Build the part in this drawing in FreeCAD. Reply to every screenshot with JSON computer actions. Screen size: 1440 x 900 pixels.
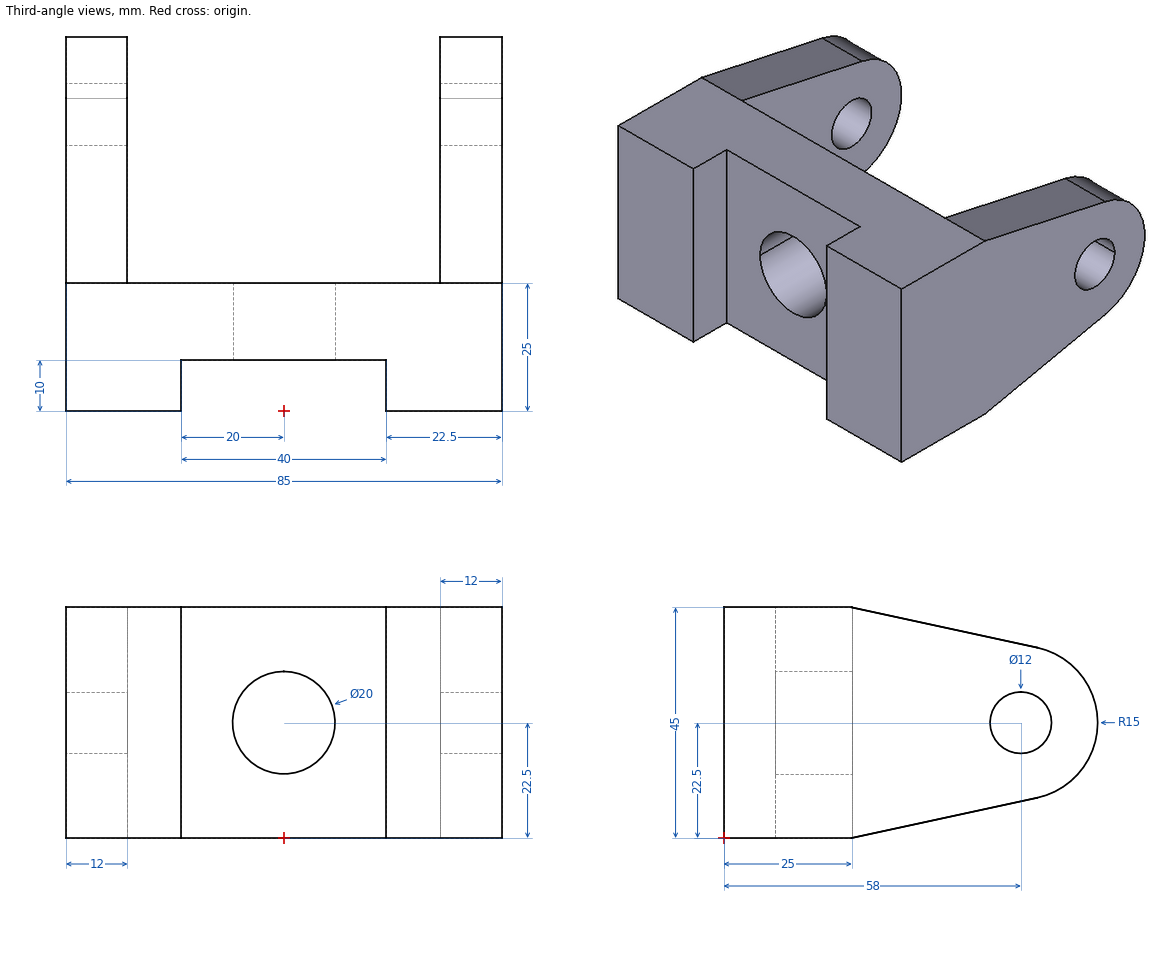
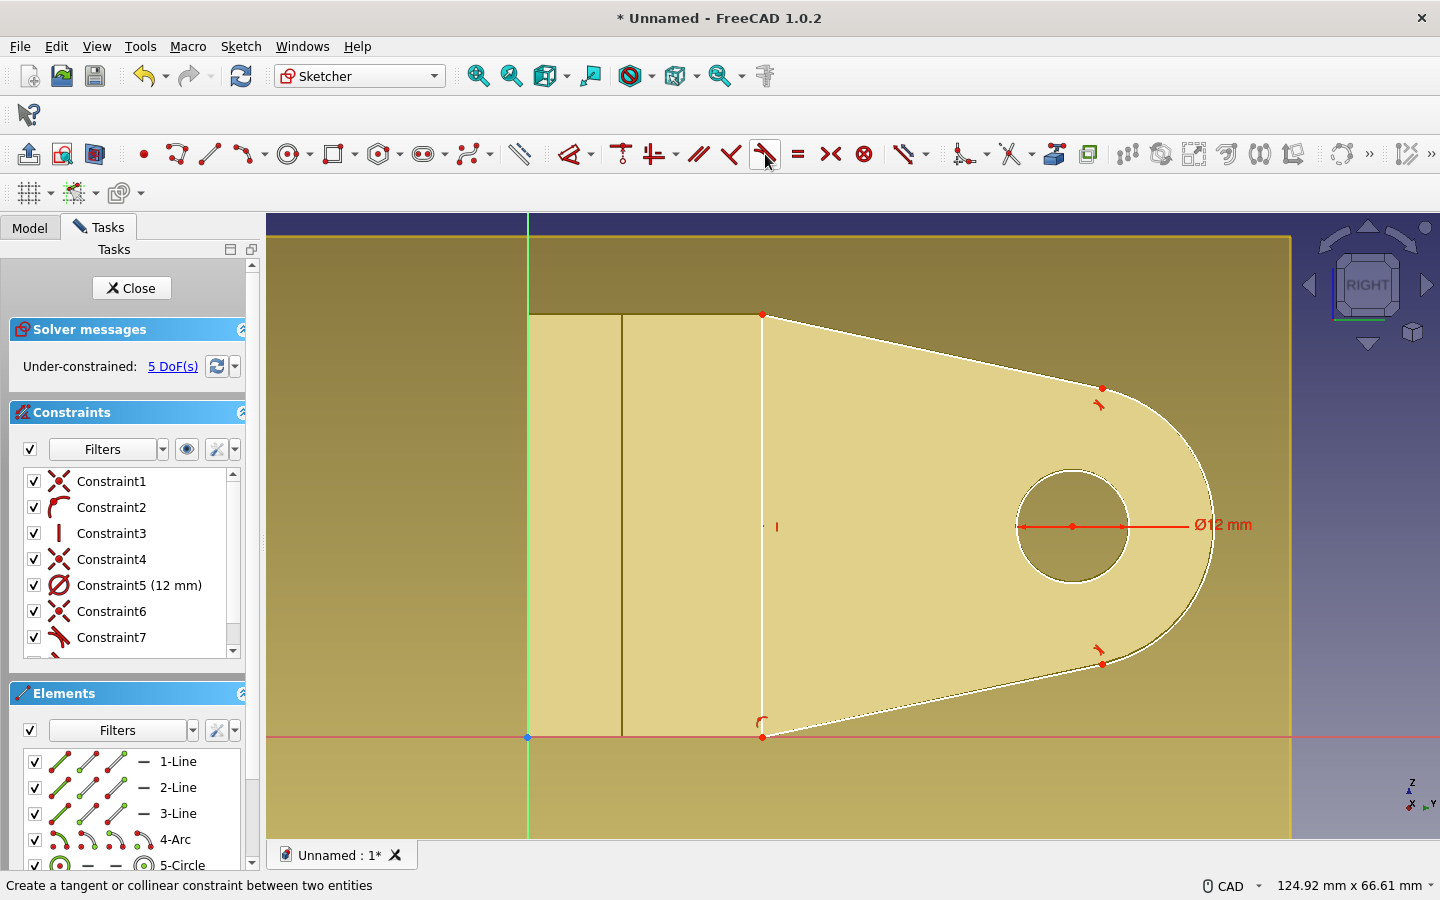
{"action": "key", "text": "d"}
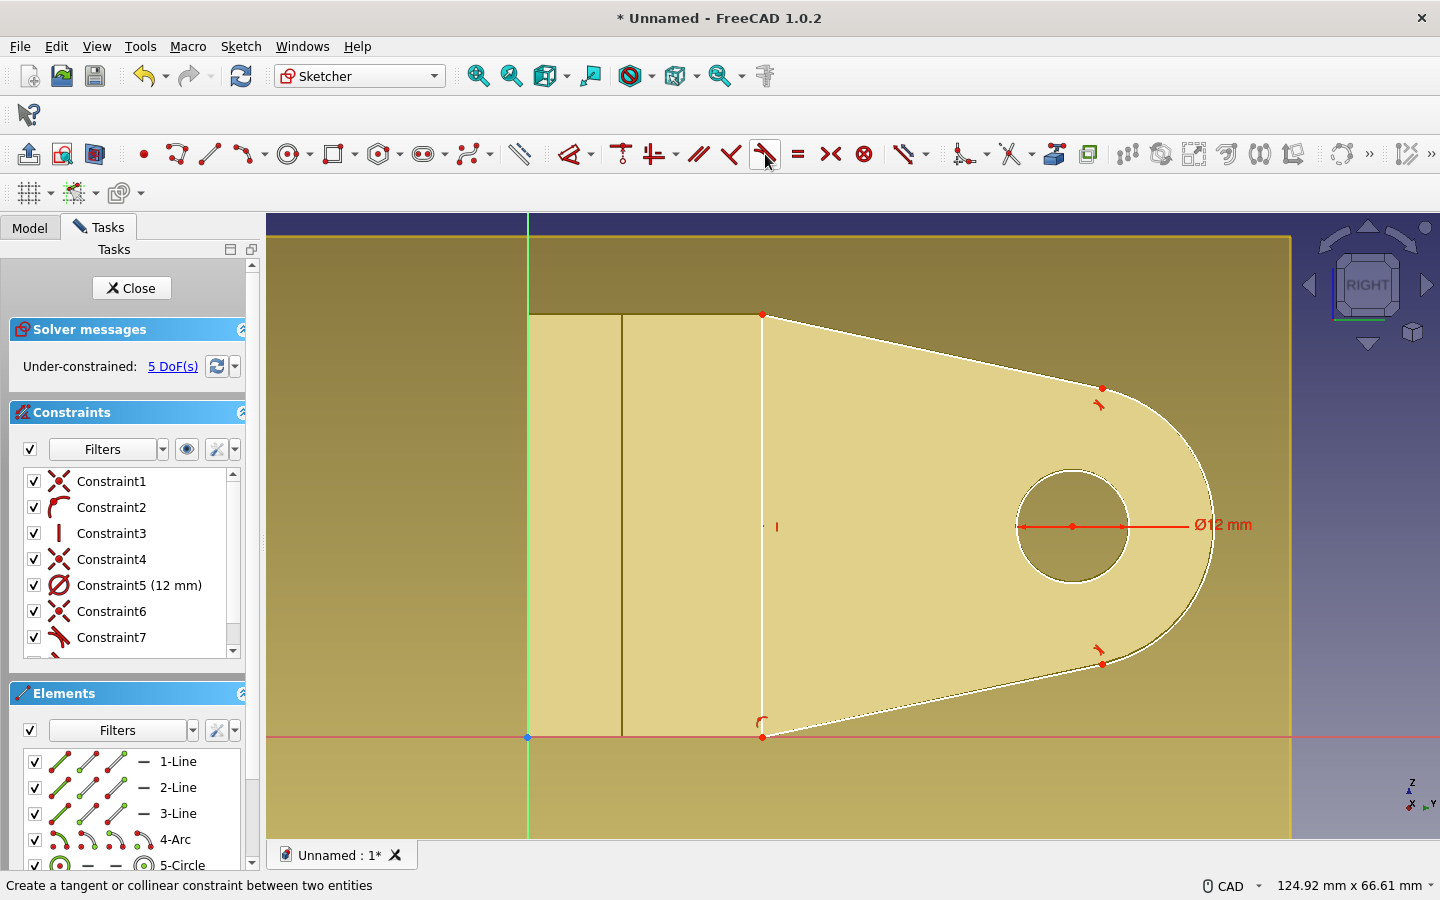
{"action": "left_click", "coordinate": [1194, 600]}
{"action": "left_click", "coordinate": [1221, 617]}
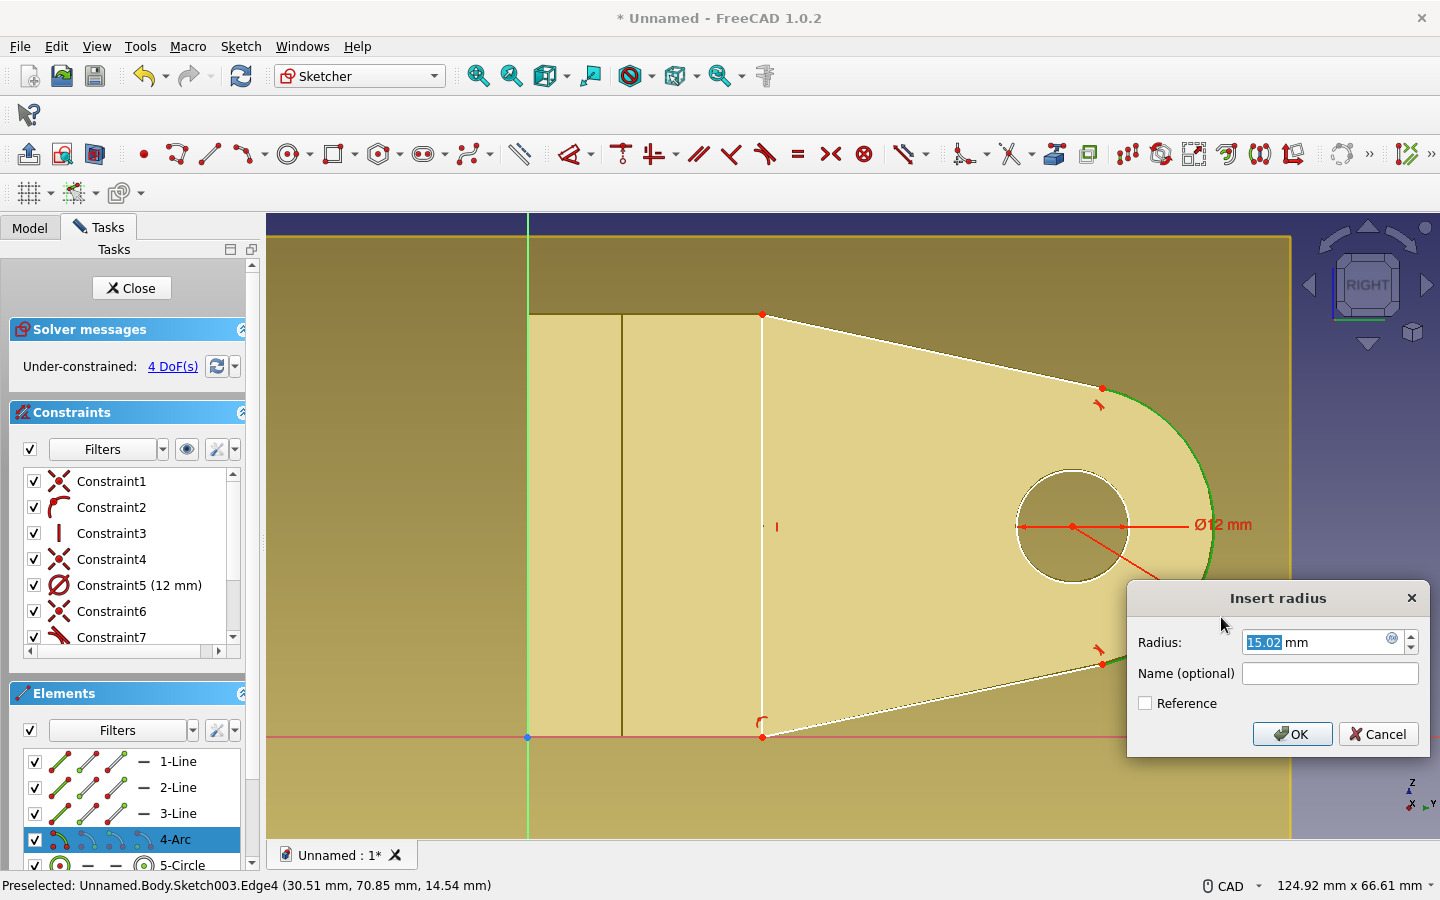
{"action": "type", "text": "15"}
{"action": "key", "text": "Return"}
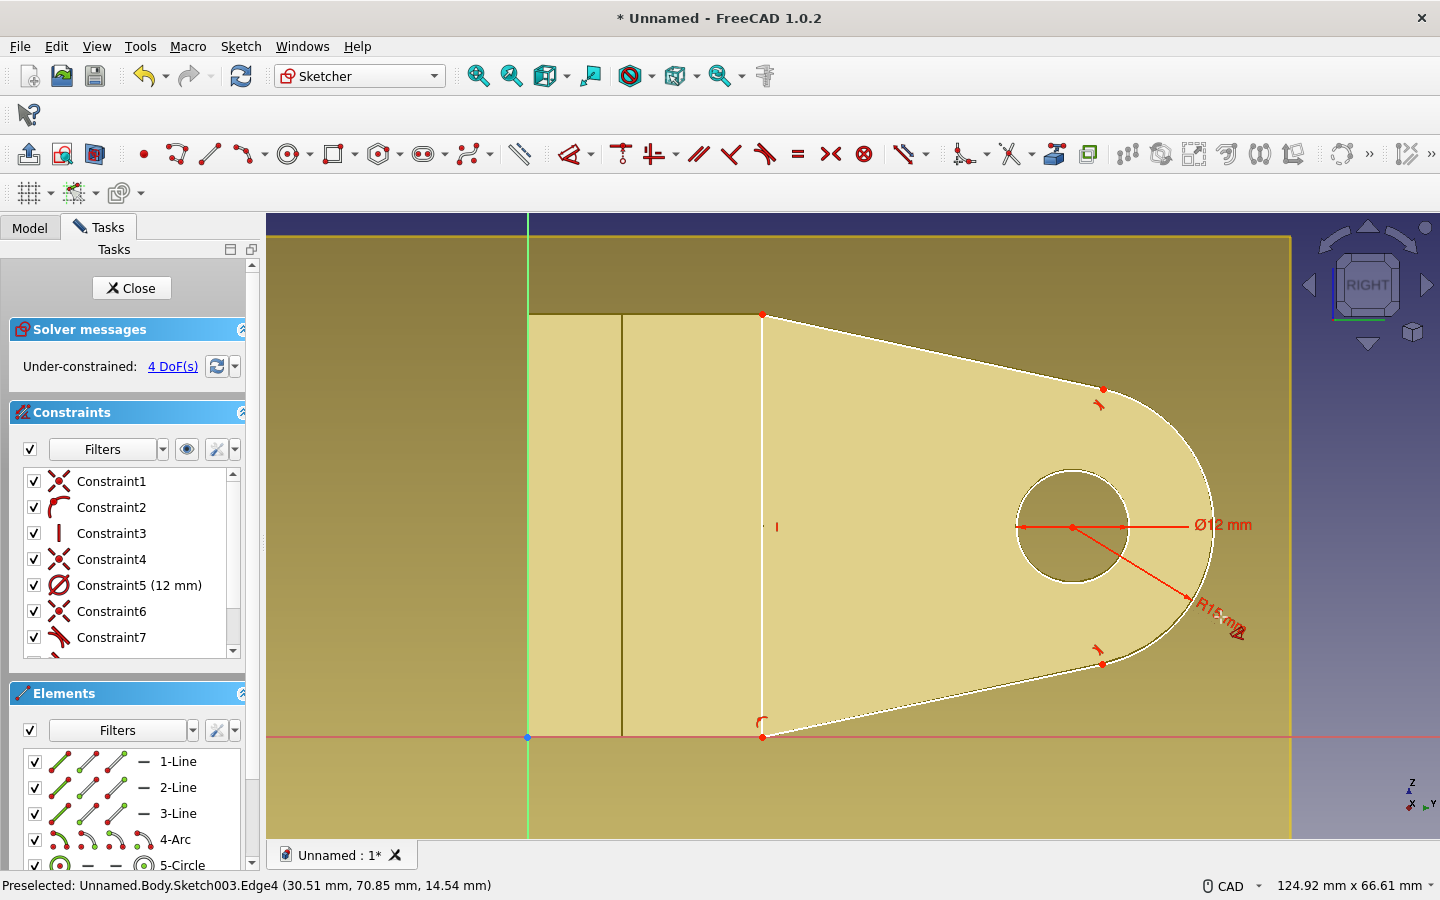
{"action": "left_click", "coordinate": [762, 442]}
{"action": "left_click", "coordinate": [728, 526]}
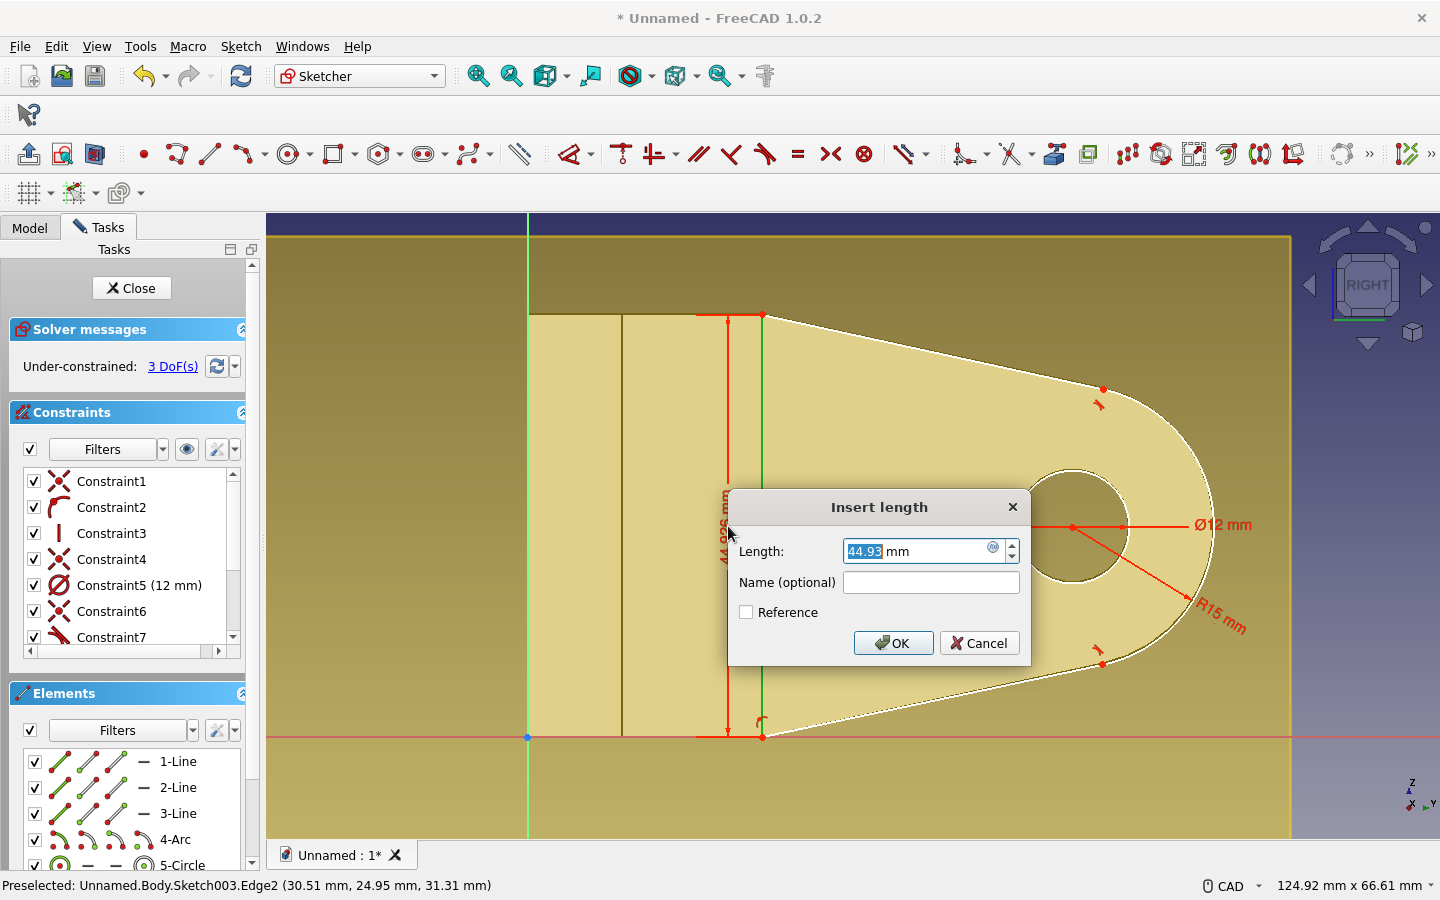
{"action": "type", "text": "45"}
{"action": "key", "text": "Return"}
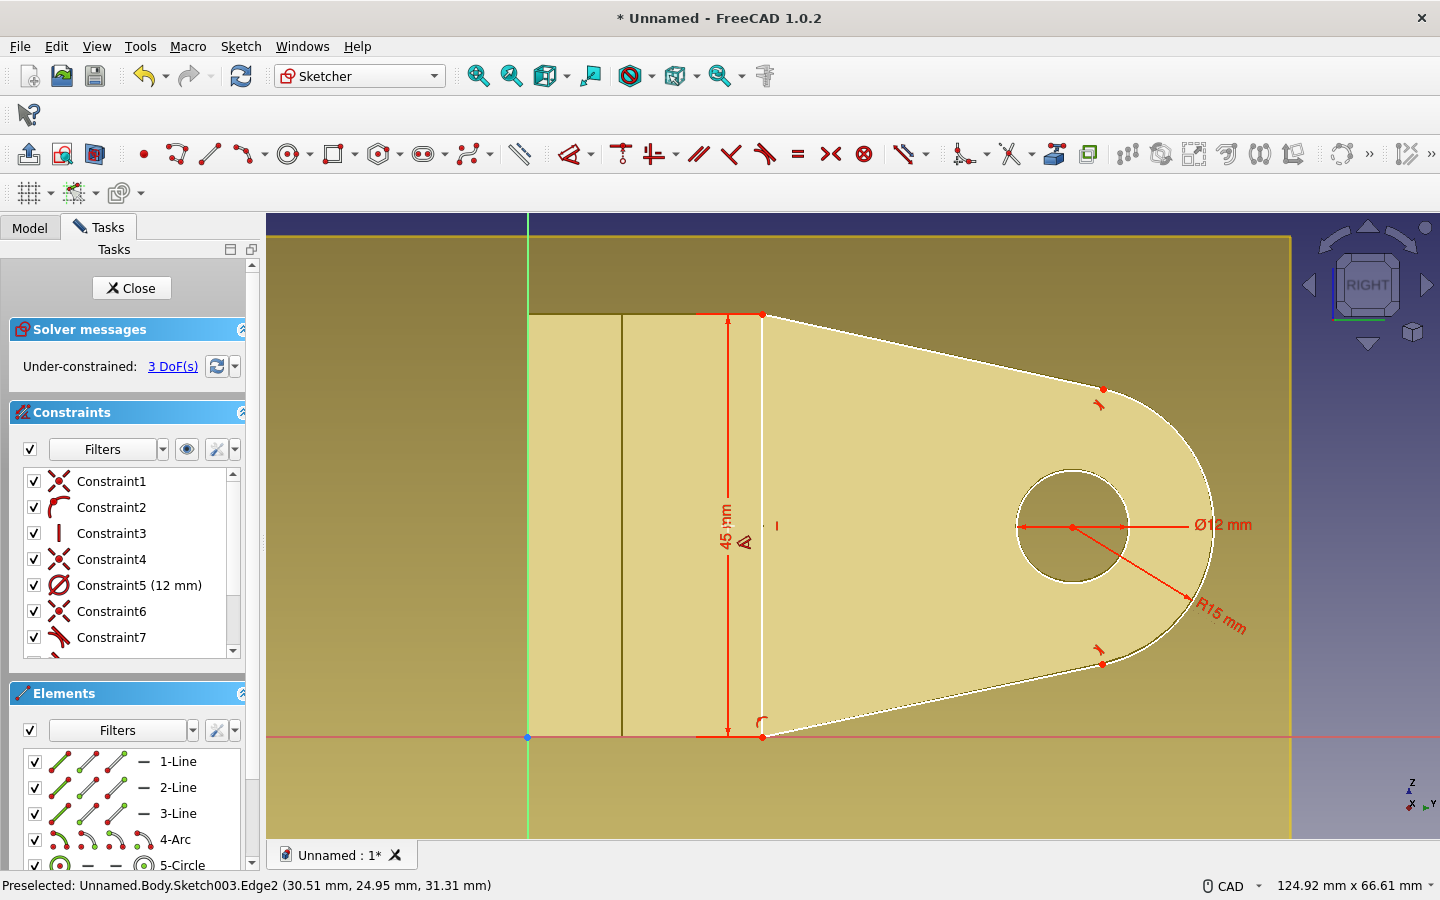
{"action": "left_click", "coordinate": [1073, 527]}
{"action": "left_click", "coordinate": [800, 771]}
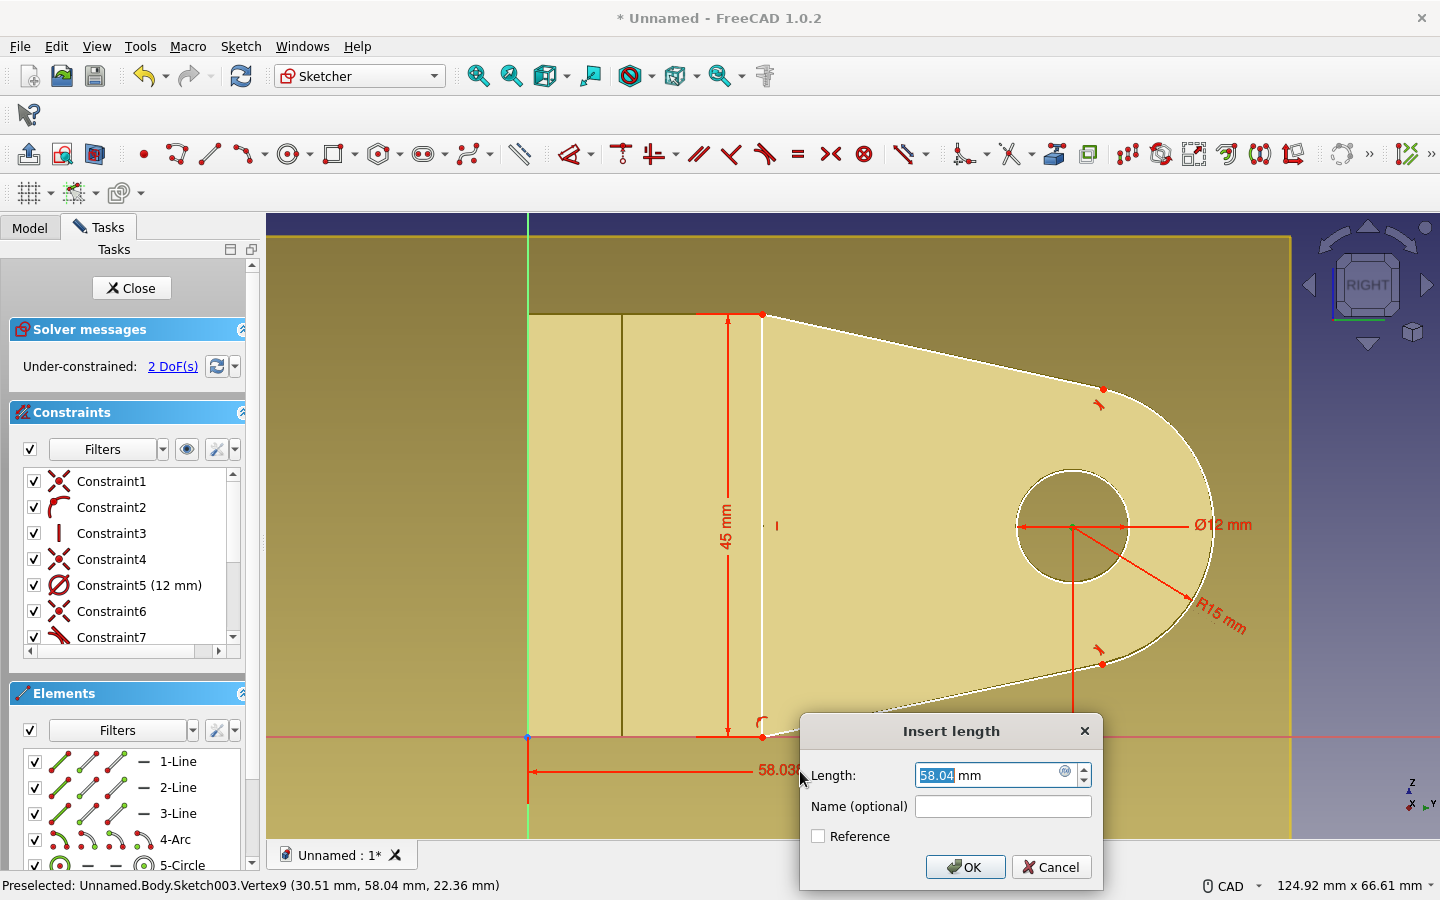
{"action": "type", "text": "58"}
{"action": "key", "text": "Return"}